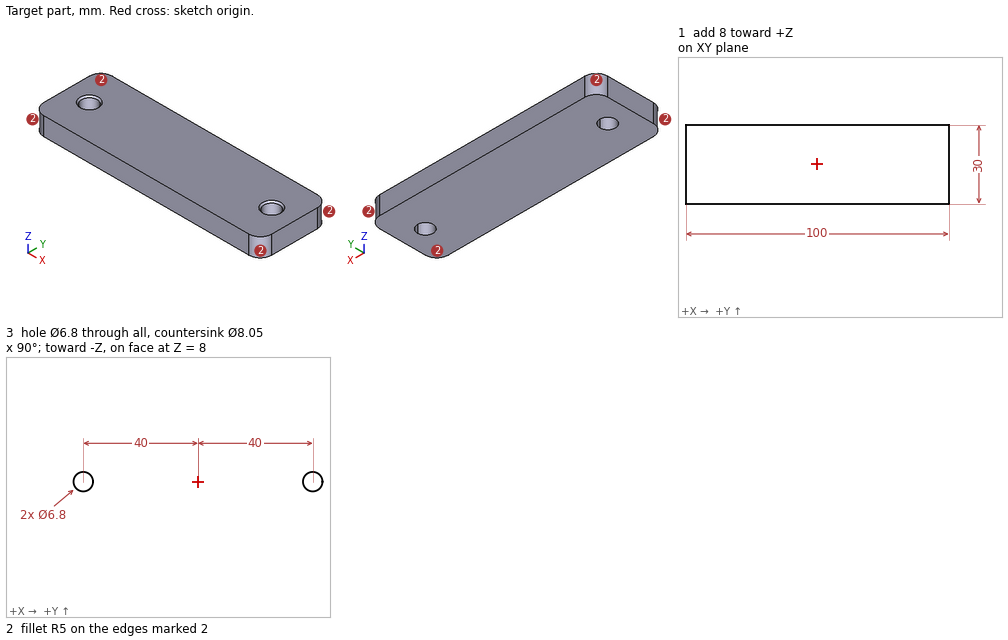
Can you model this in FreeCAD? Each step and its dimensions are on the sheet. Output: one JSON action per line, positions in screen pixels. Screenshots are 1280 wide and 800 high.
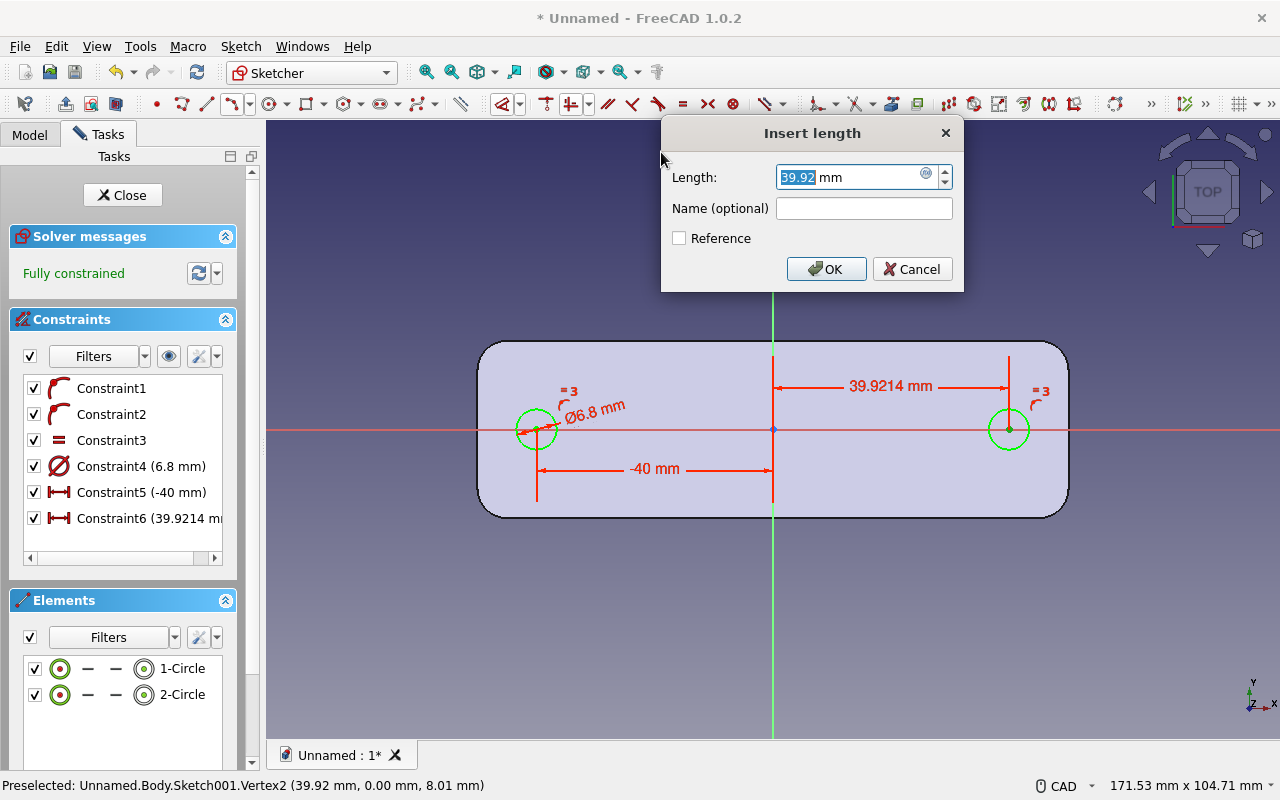
{"action": "type", "text": "40"}
{"action": "key", "text": "Return"}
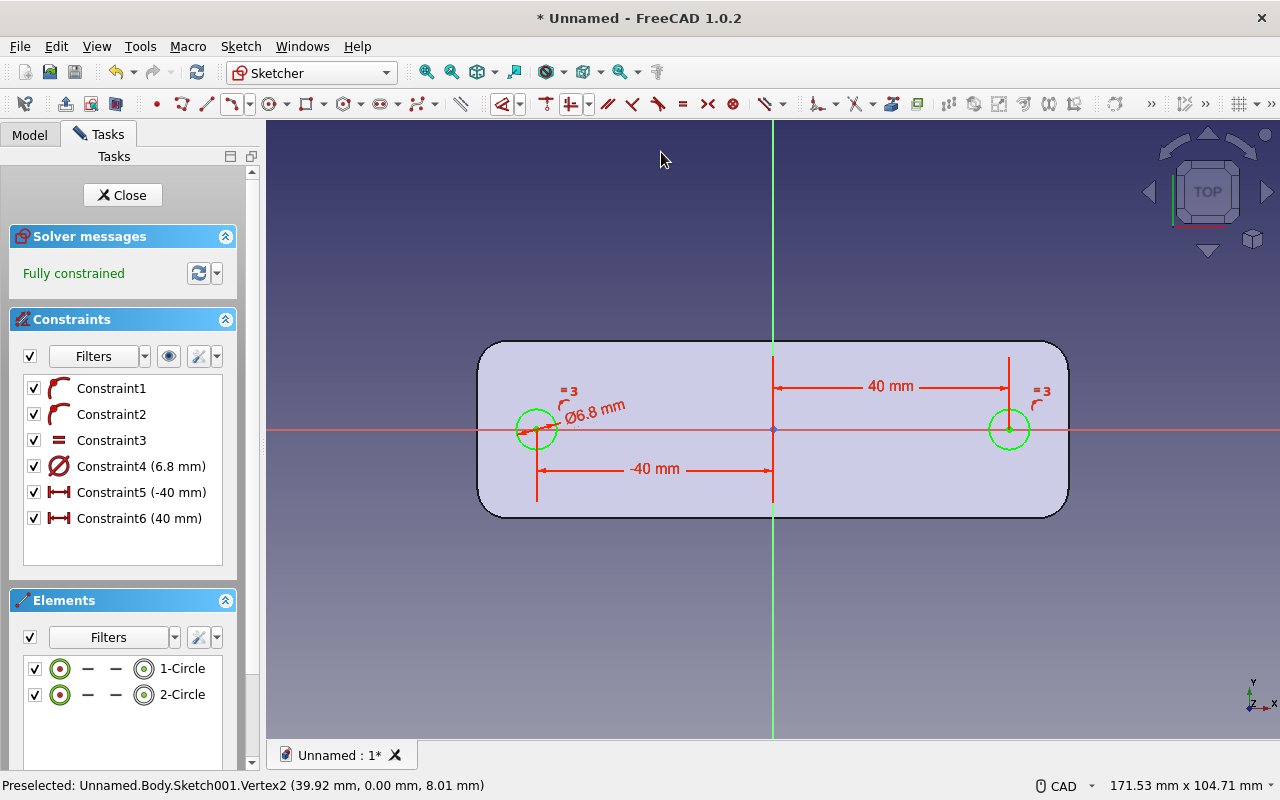
{"action": "left_click", "coordinate": [123, 195]}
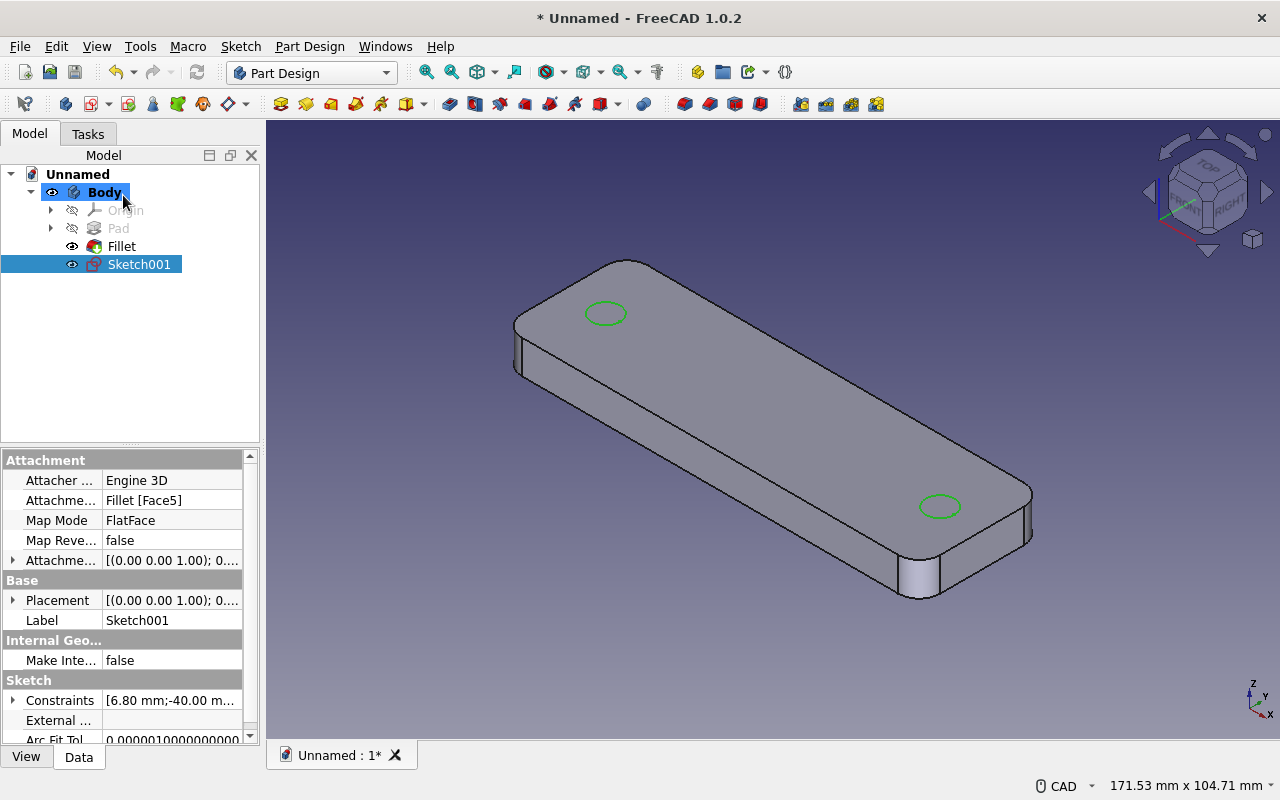
{"action": "left_click", "coordinate": [475, 104]}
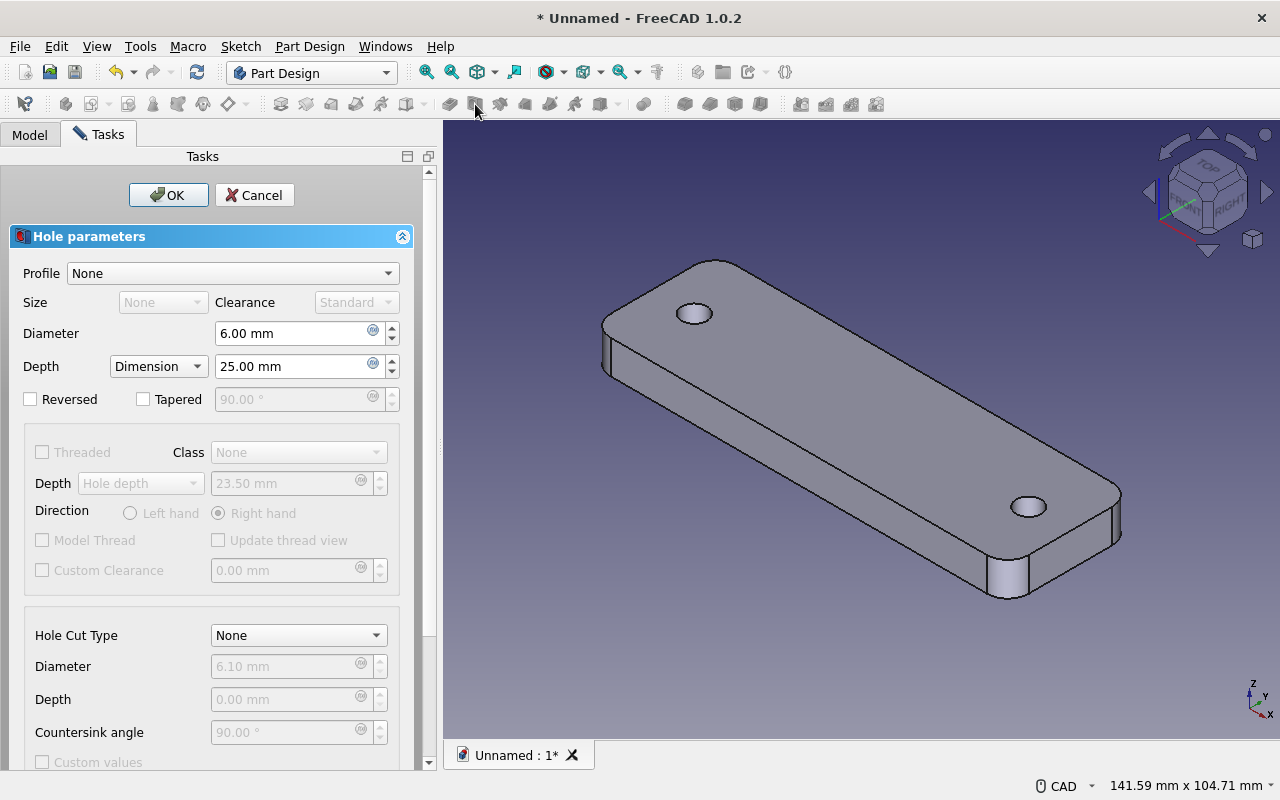
{"action": "triple_click", "coordinate": [300, 334]}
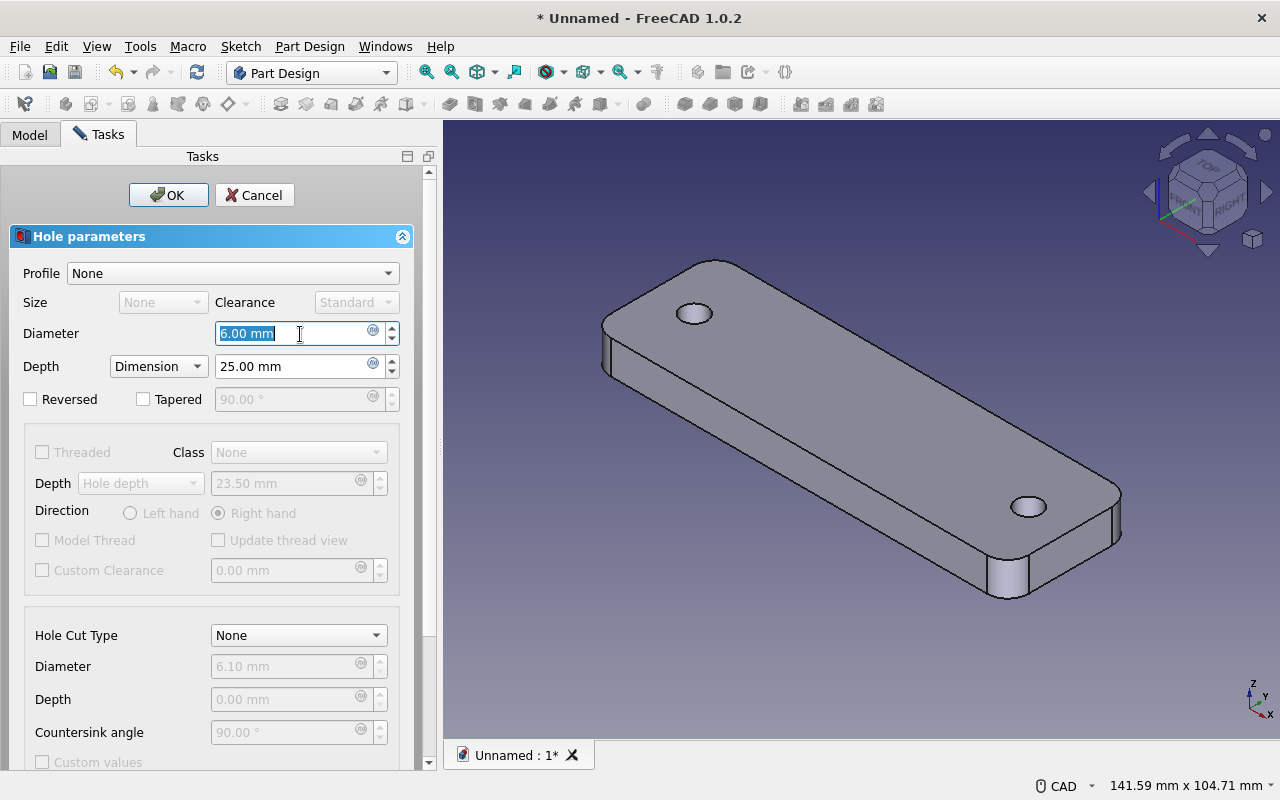
{"action": "type", "text": "6.8"}
{"action": "key", "text": "Tab"}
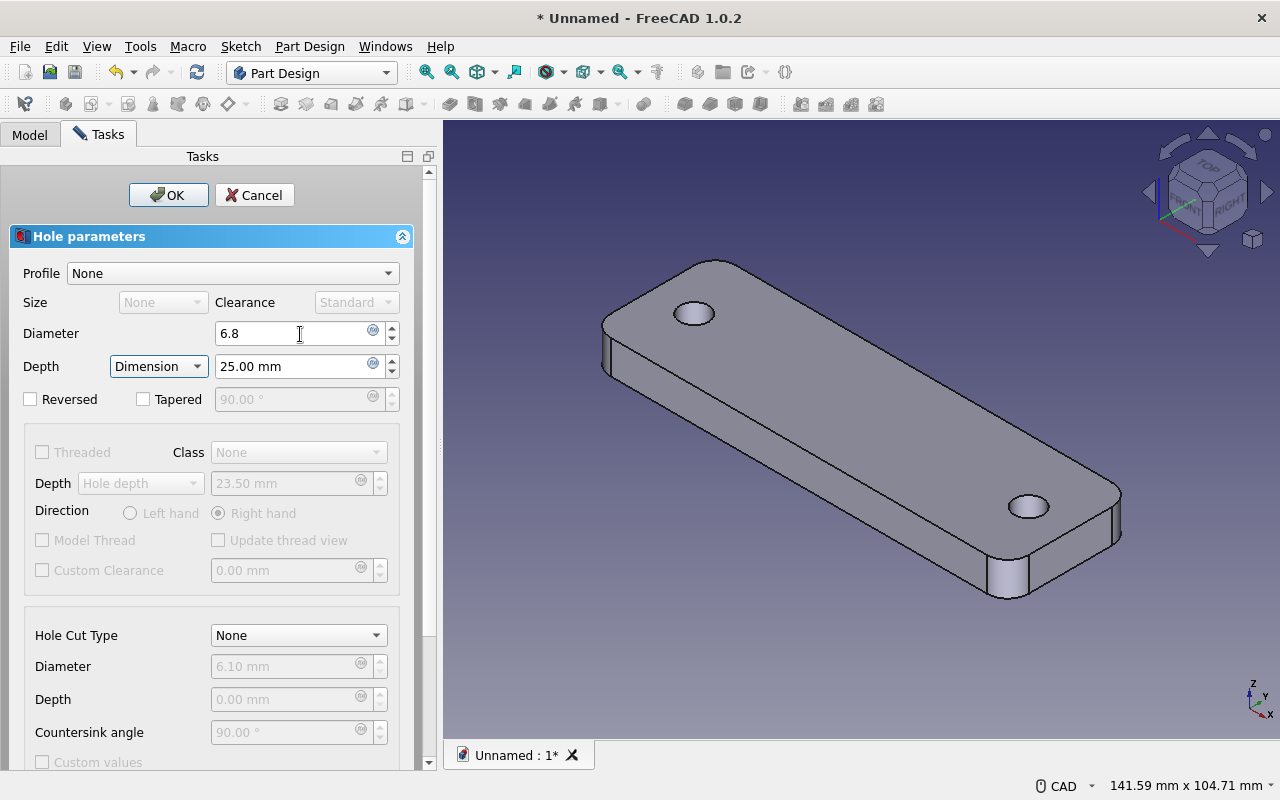
{"action": "left_click", "coordinate": [160, 366]}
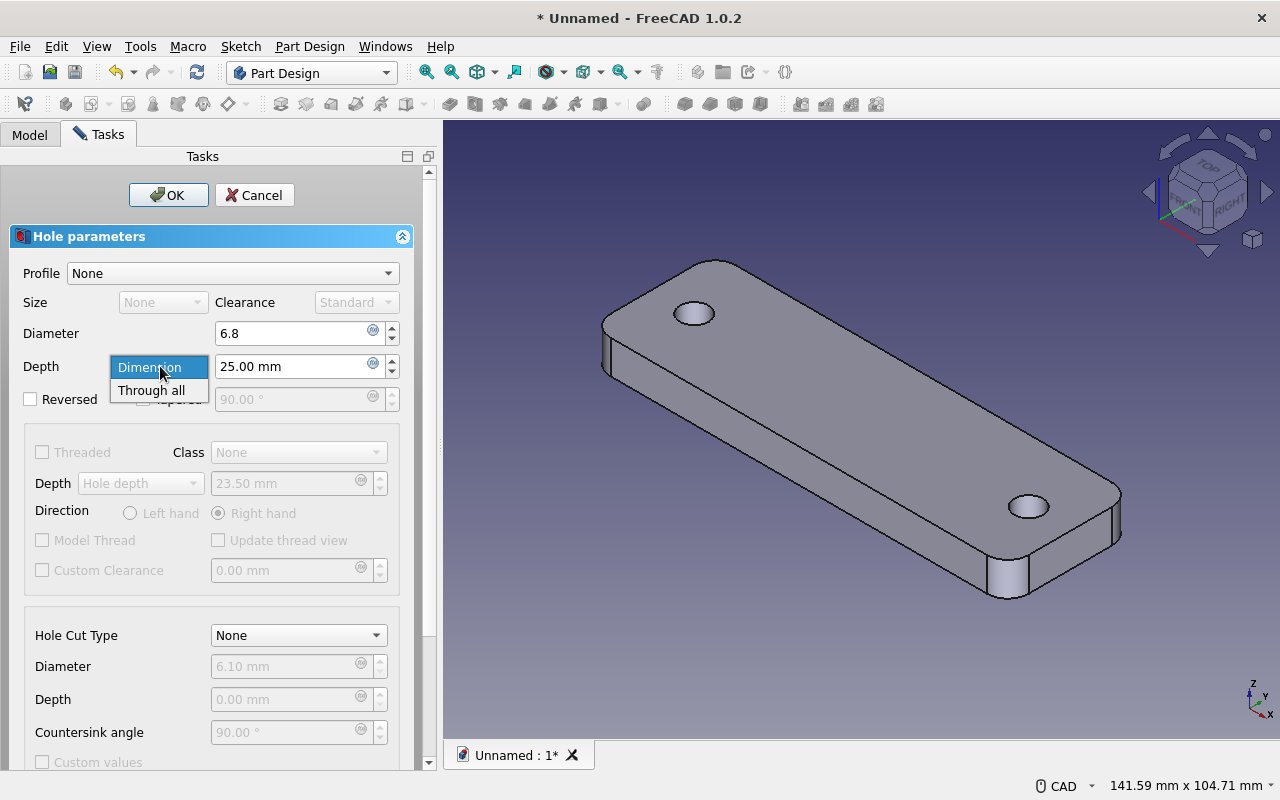
{"action": "left_click", "coordinate": [158, 390]}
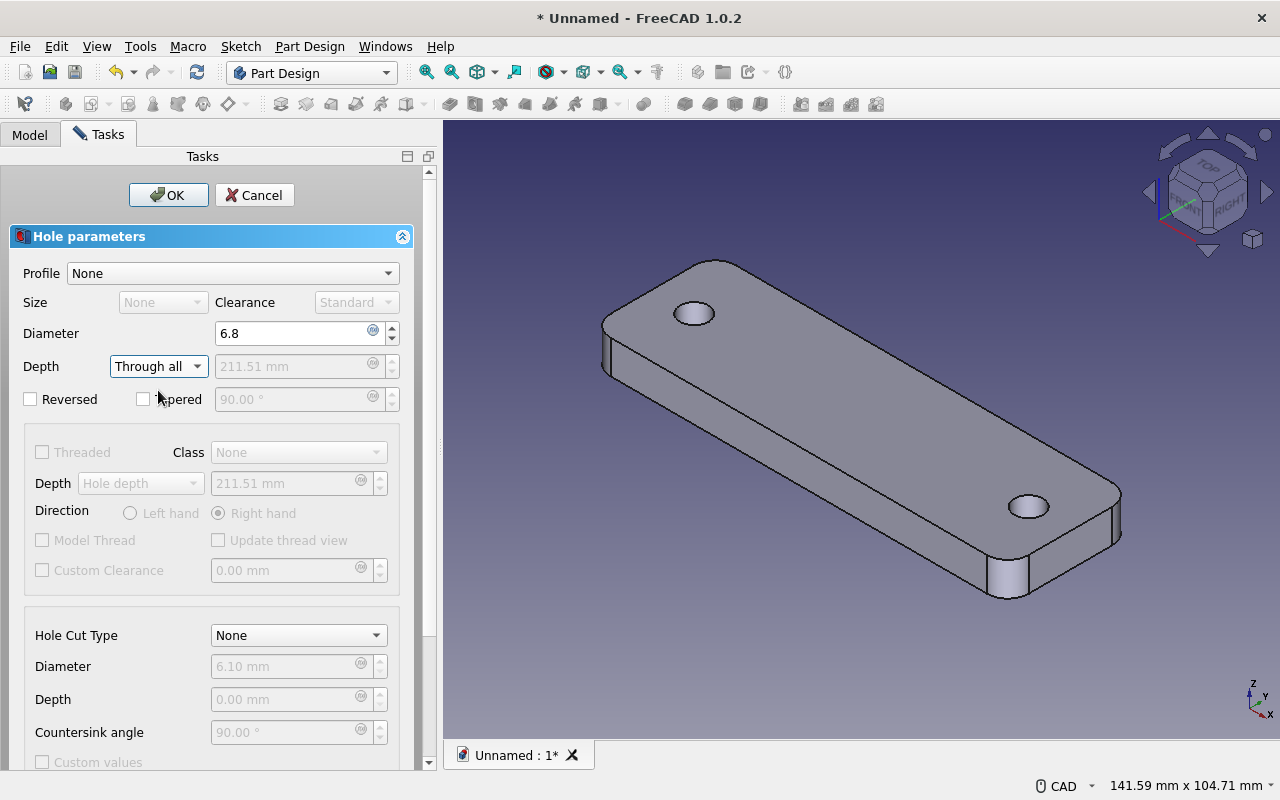
{"action": "left_click", "coordinate": [300, 636]}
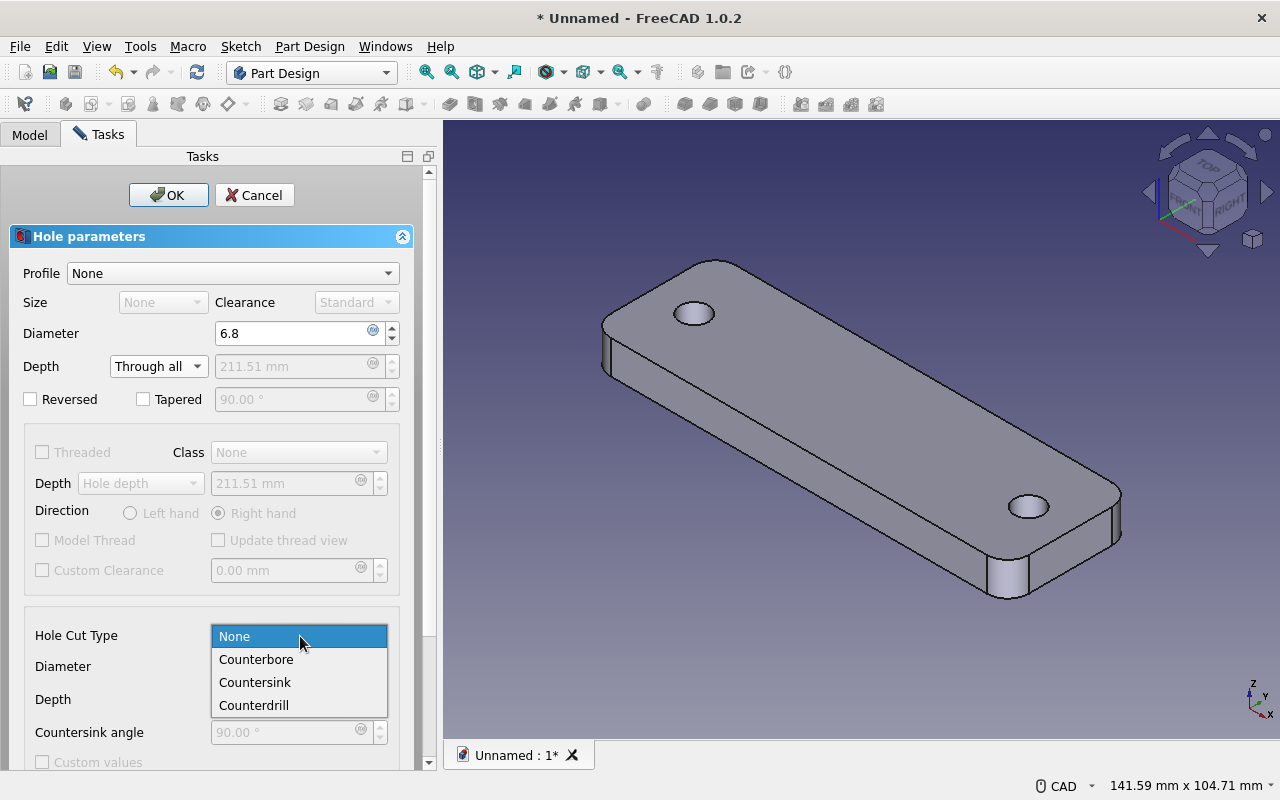
{"action": "left_click", "coordinate": [298, 682]}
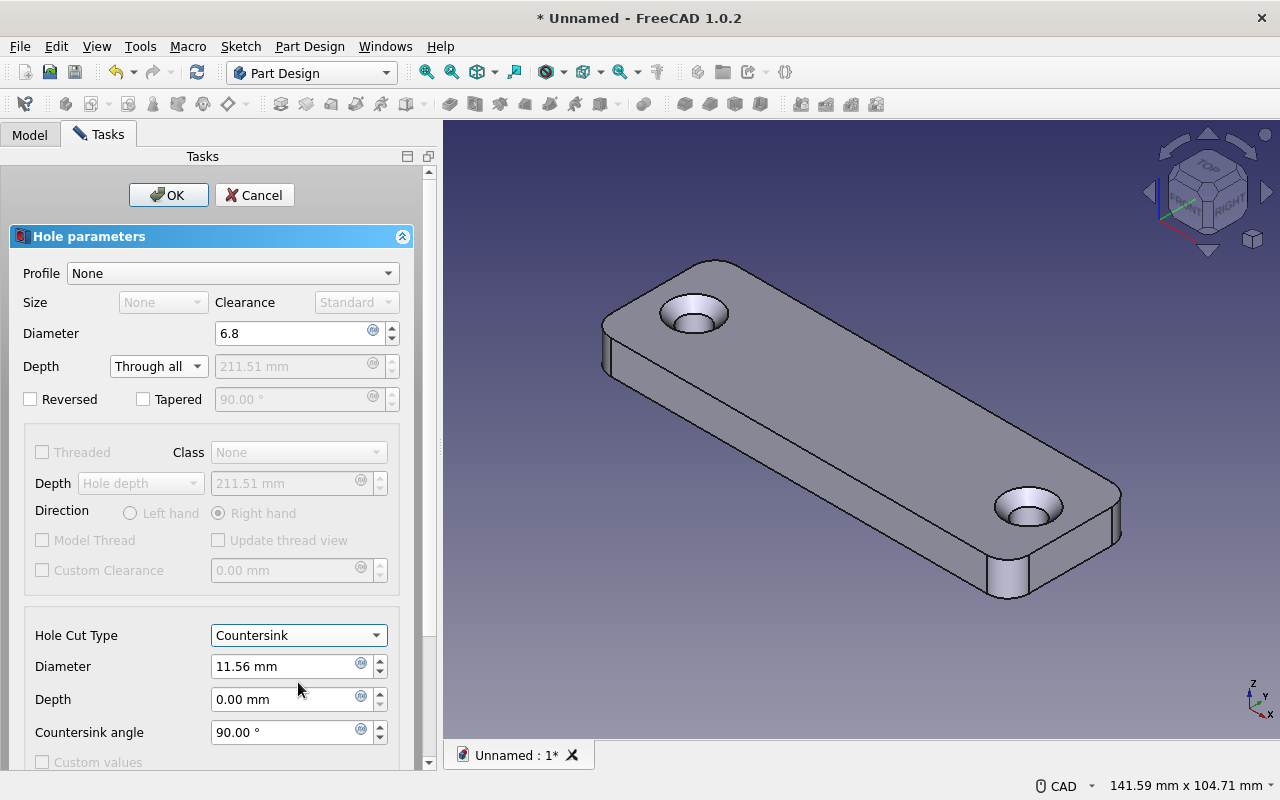
{"action": "triple_click", "coordinate": [292, 666]}